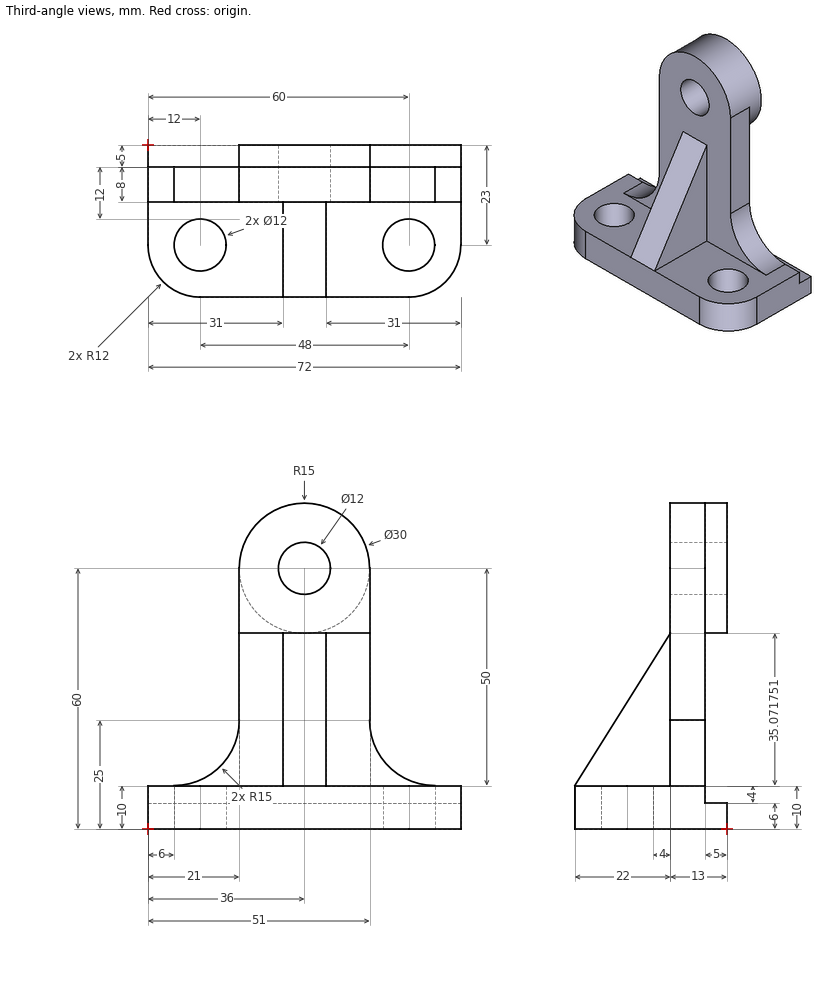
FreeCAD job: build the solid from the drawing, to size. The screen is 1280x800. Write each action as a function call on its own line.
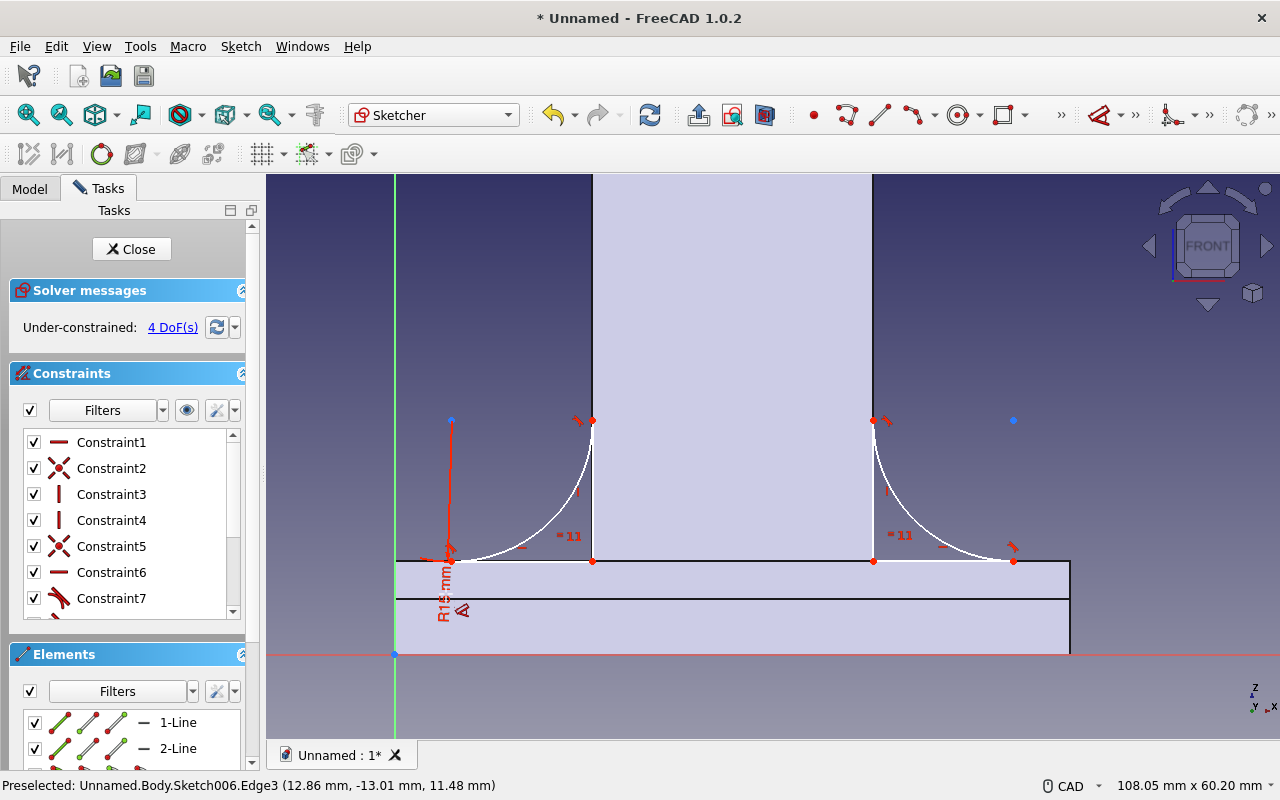
click(452, 562)
click(423, 689)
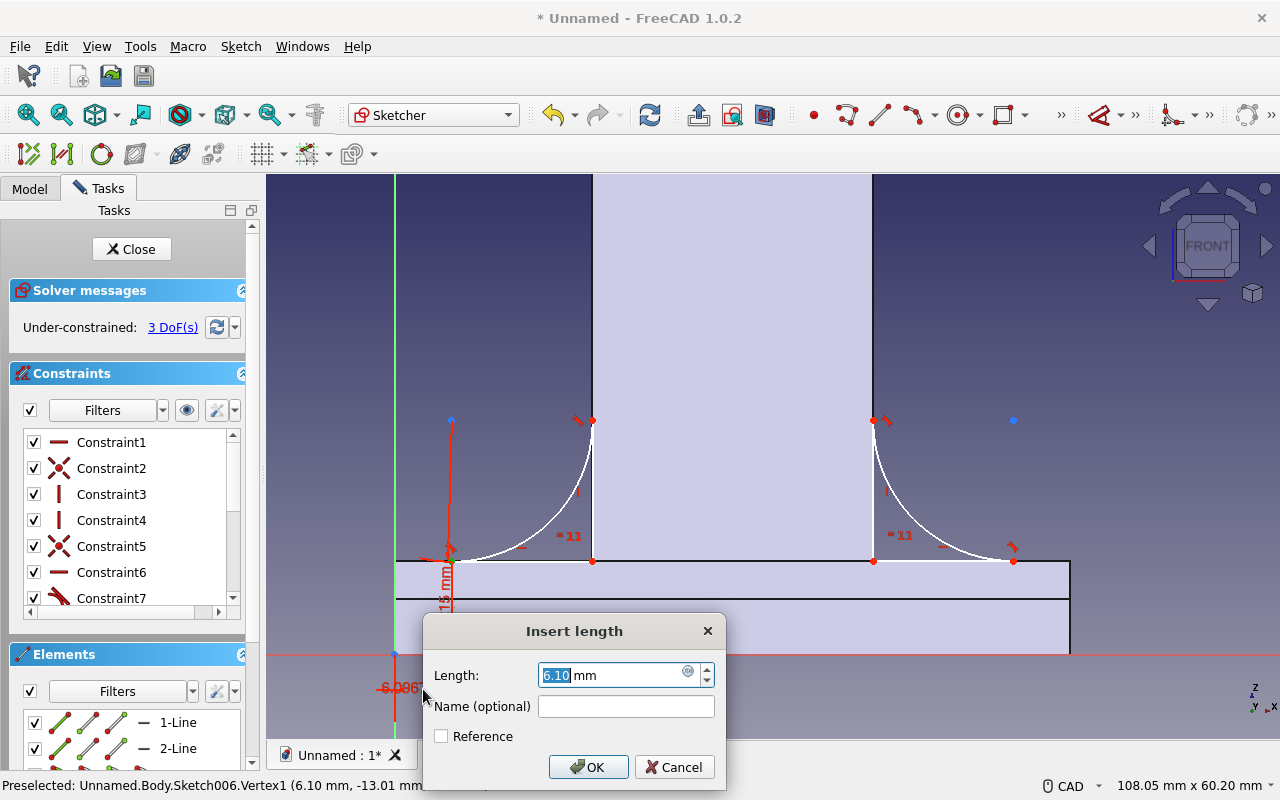
text(6)
key(Return)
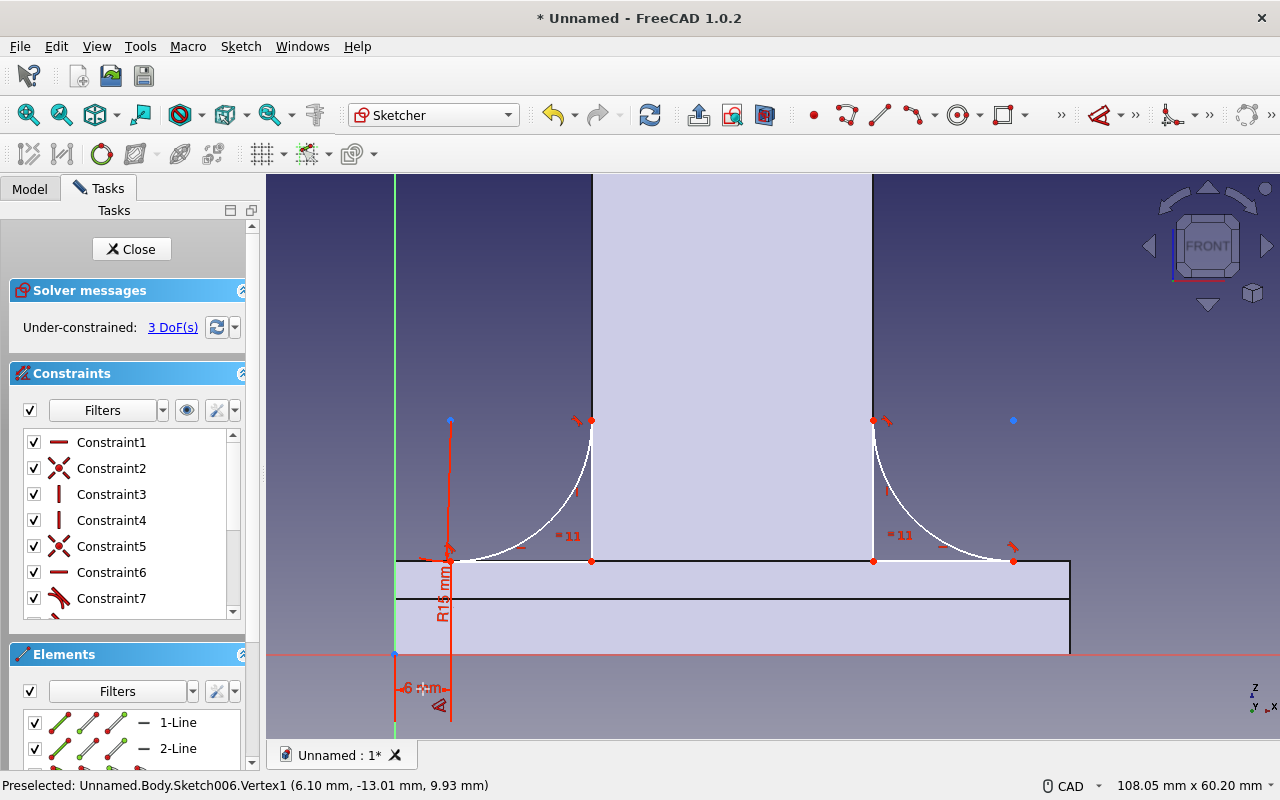
click(451, 562)
click(361, 608)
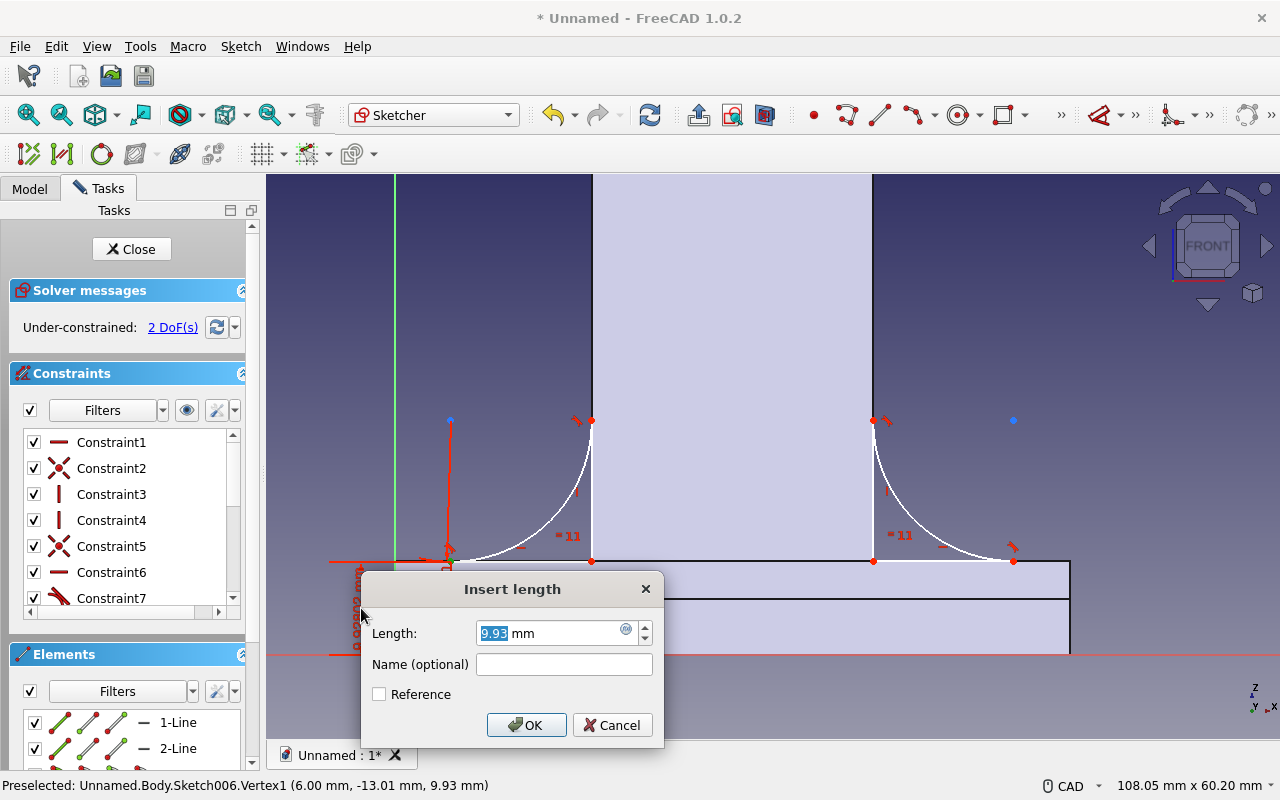
text(10)
key(Return)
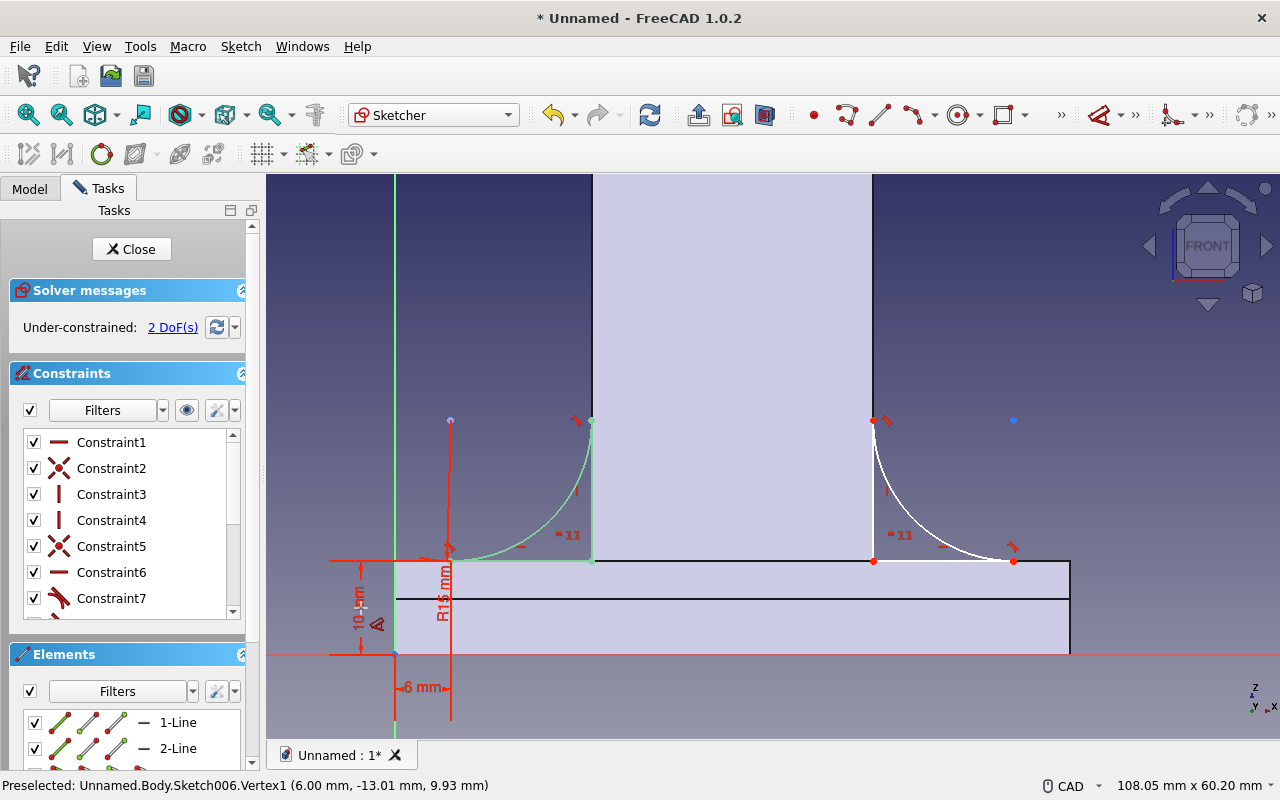
click(873, 420)
click(634, 386)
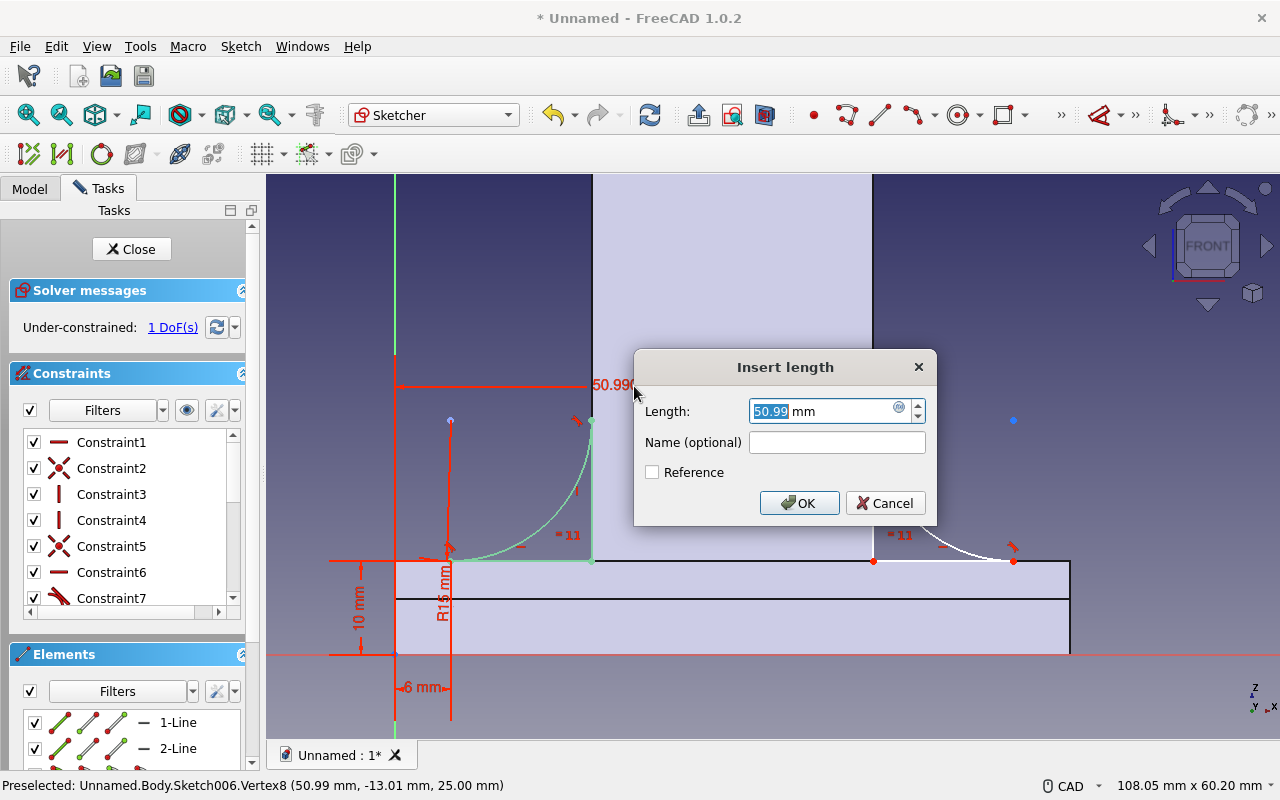
text(51)
key(Return)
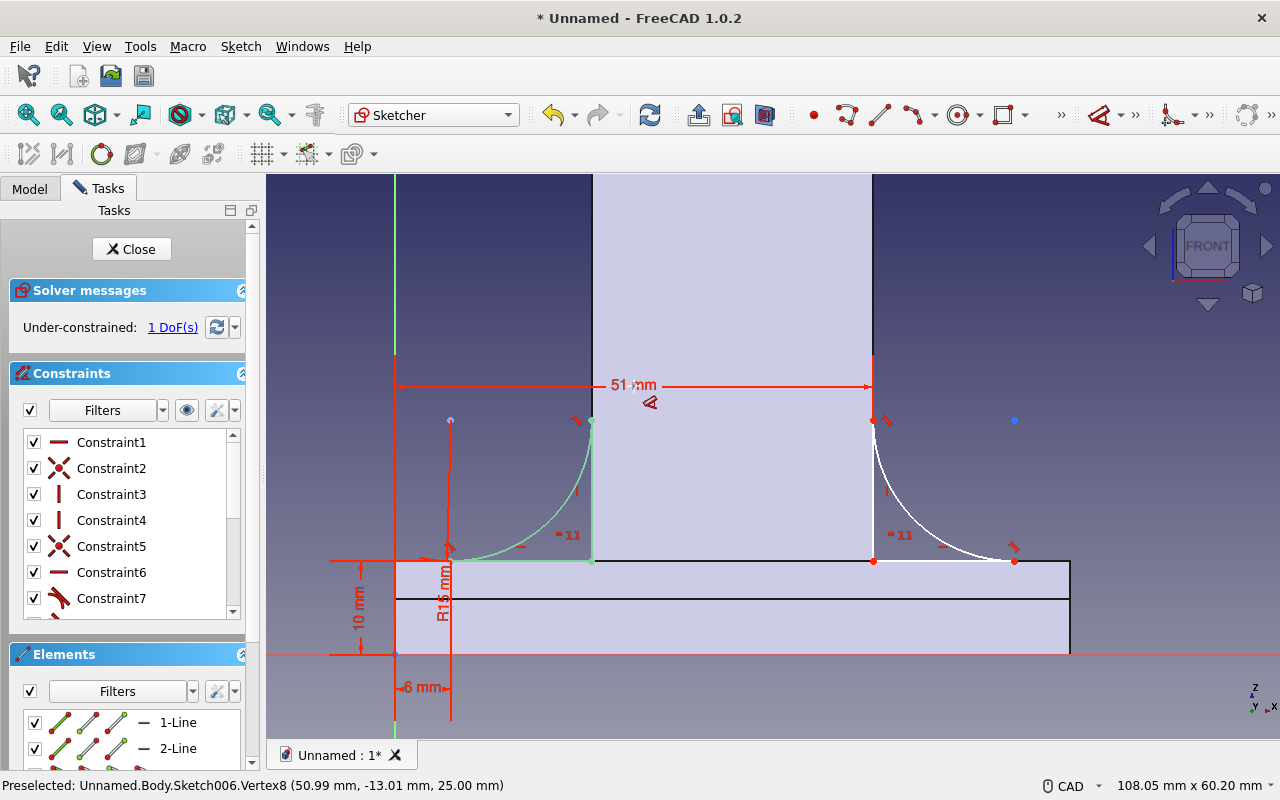
click(873, 420)
click(361, 538)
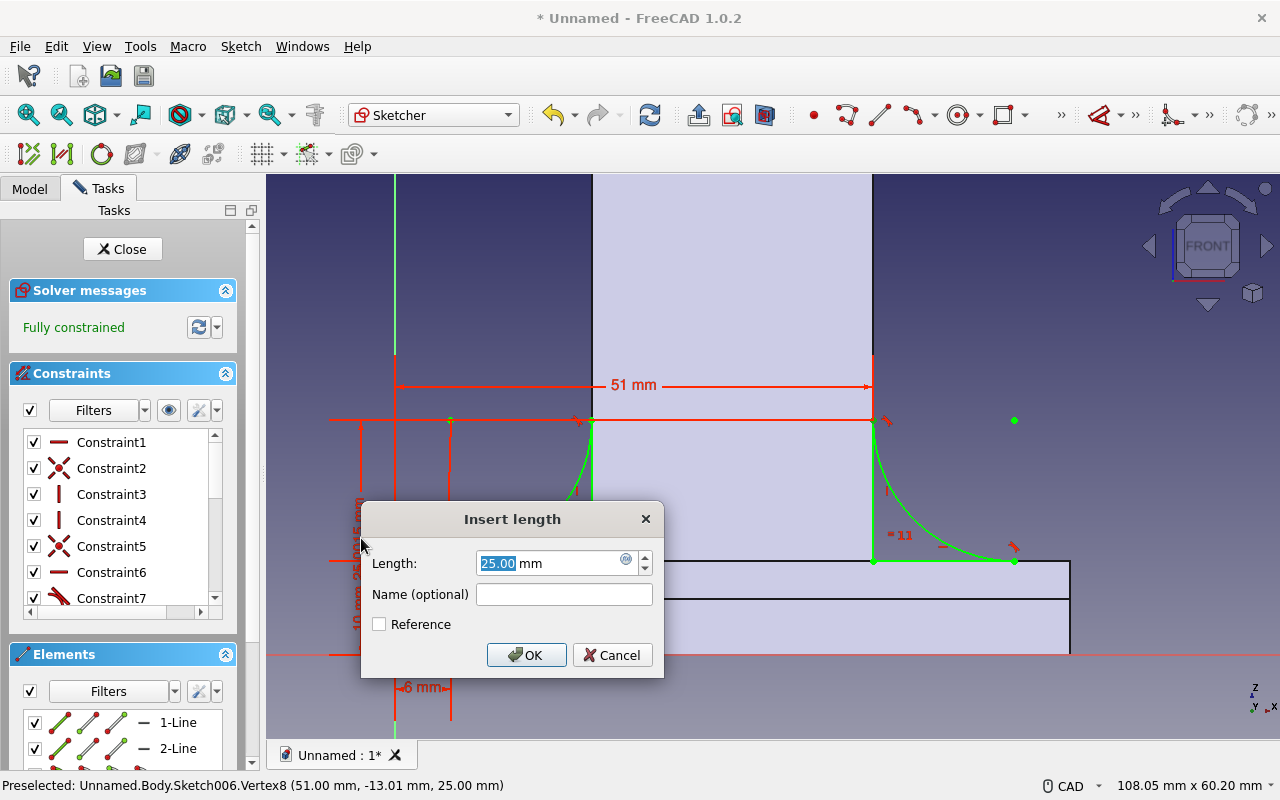
text(25)
key(Return)
key(Escape)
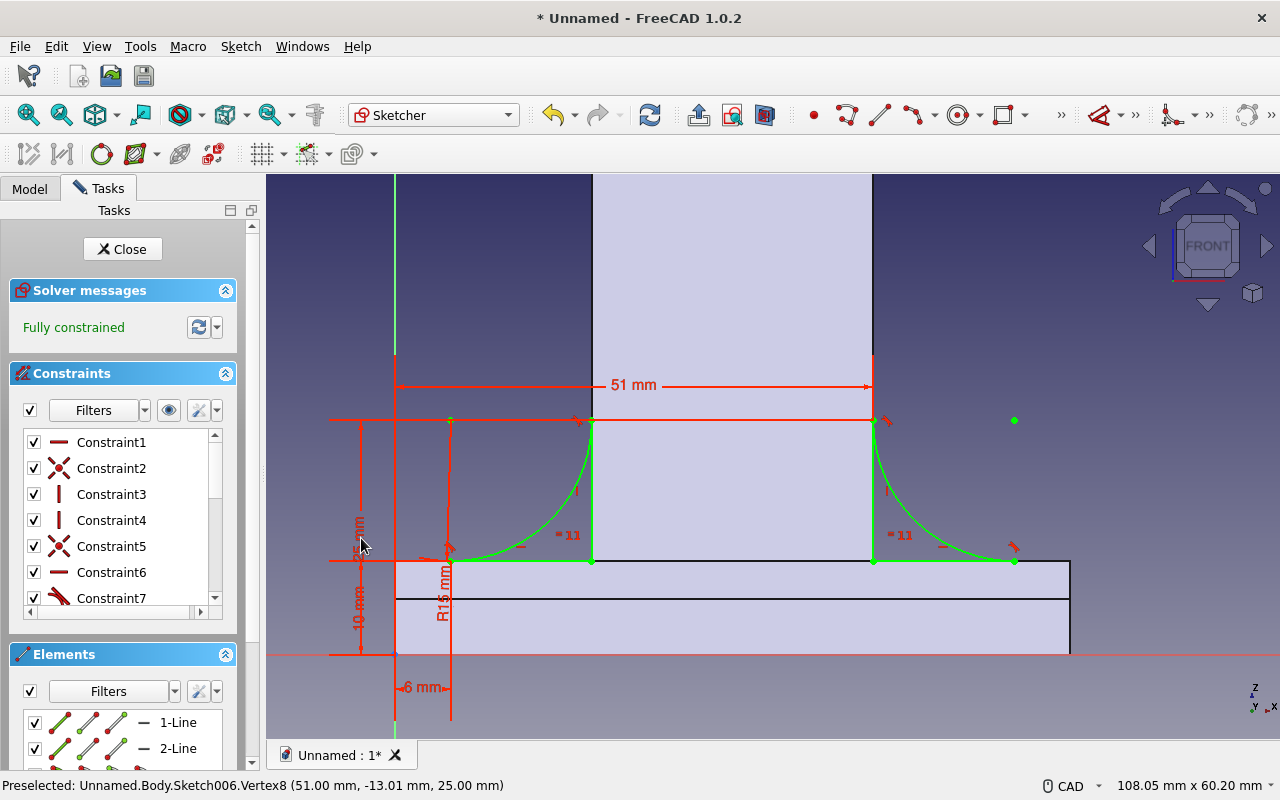
click(123, 249)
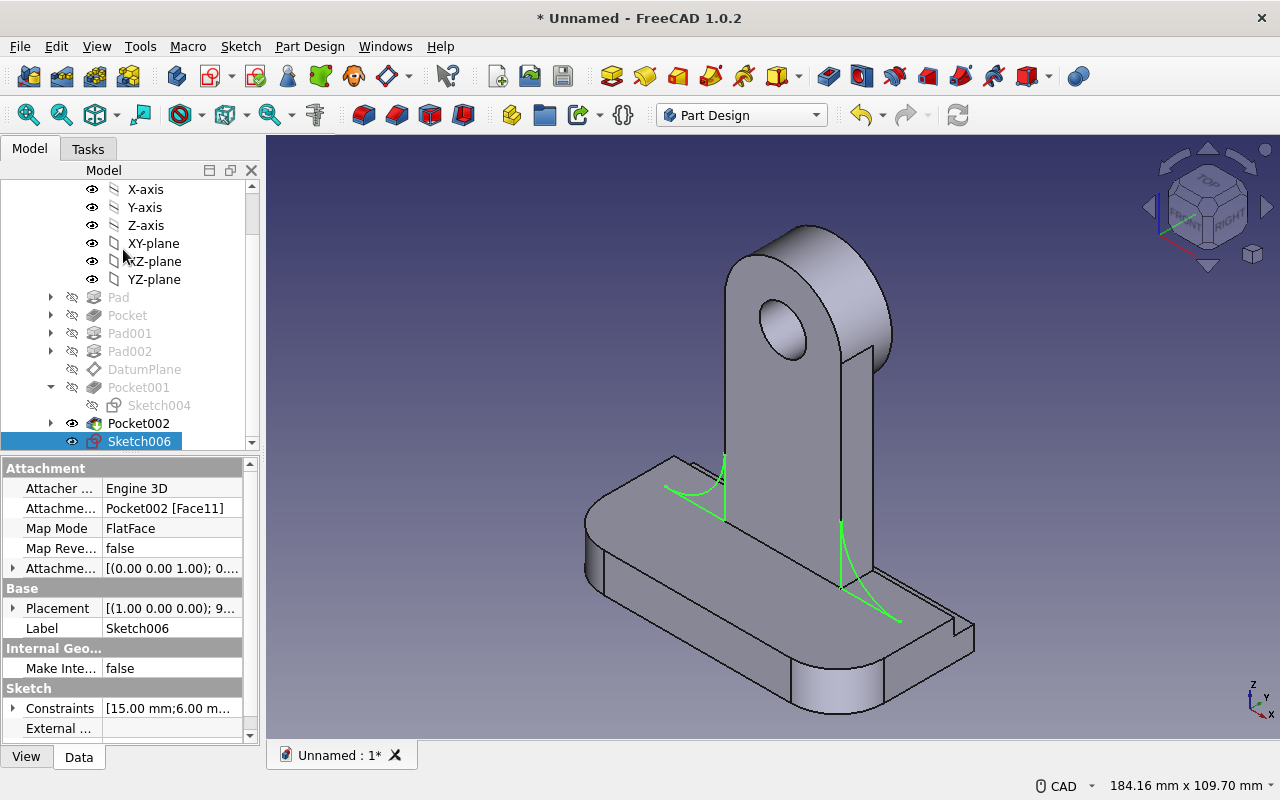
click(612, 76)